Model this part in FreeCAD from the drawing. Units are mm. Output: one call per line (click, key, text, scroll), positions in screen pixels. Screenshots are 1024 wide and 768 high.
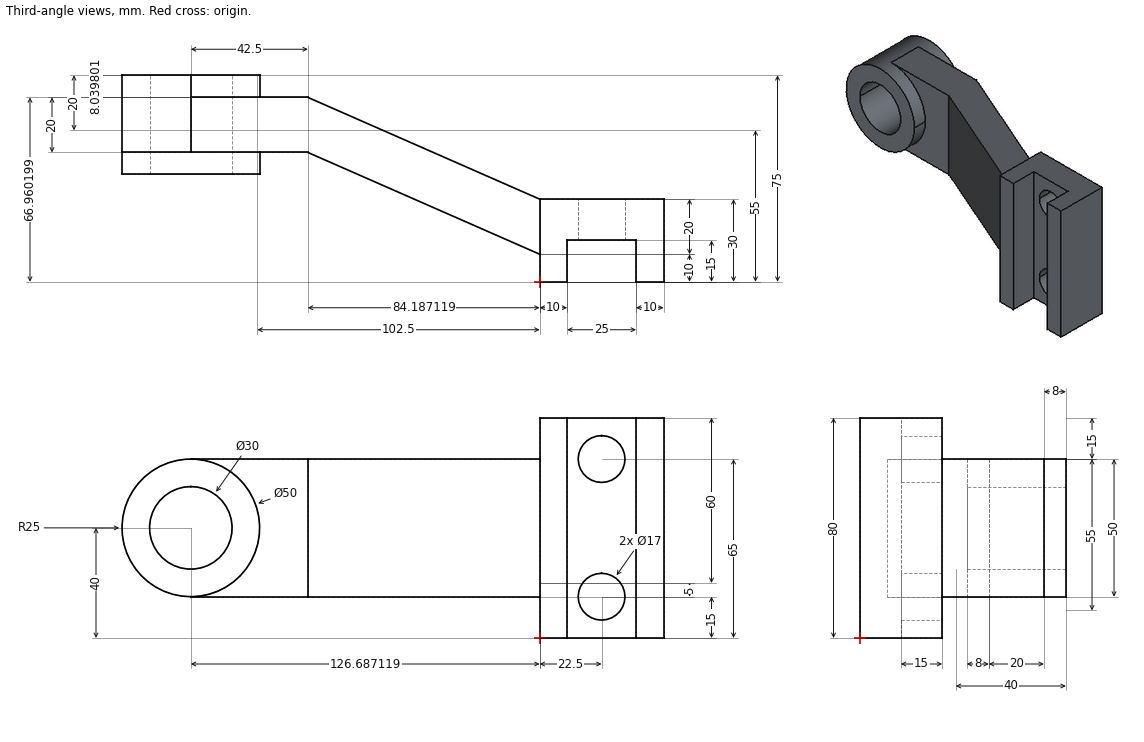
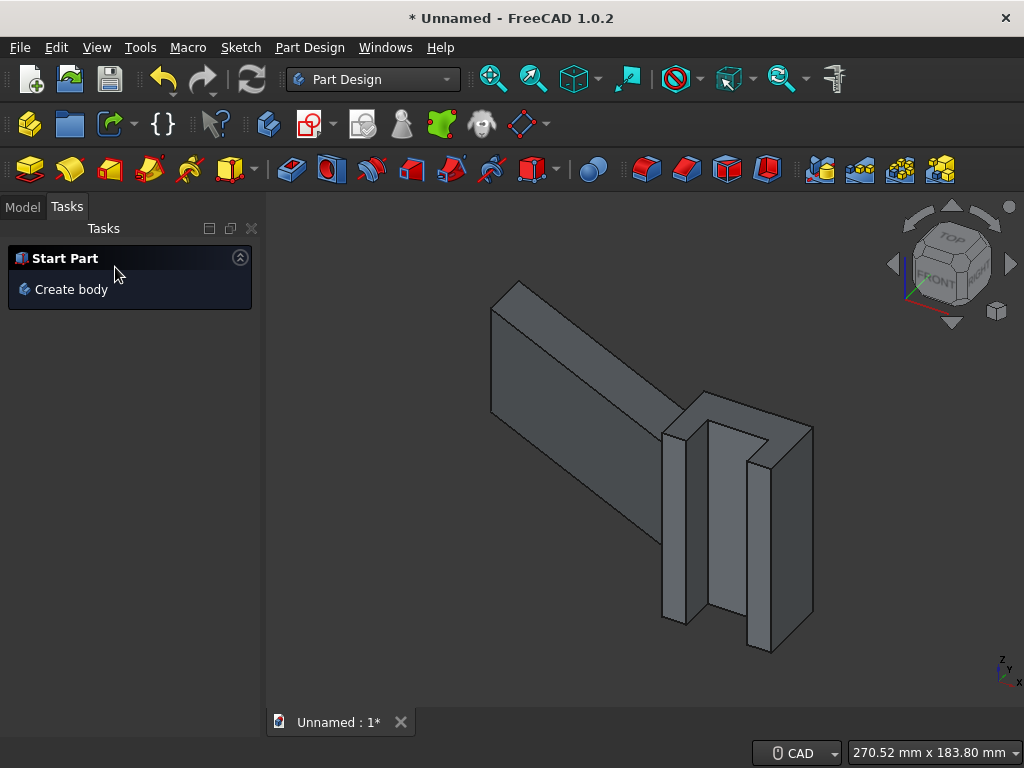
key(5)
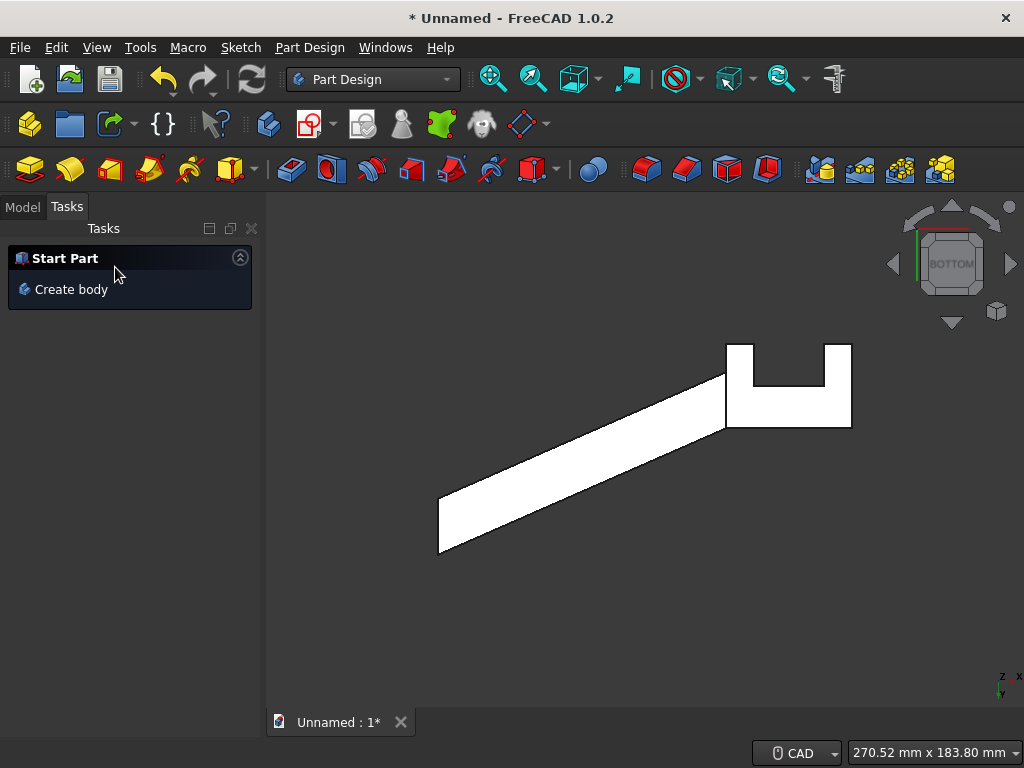
click(582, 463)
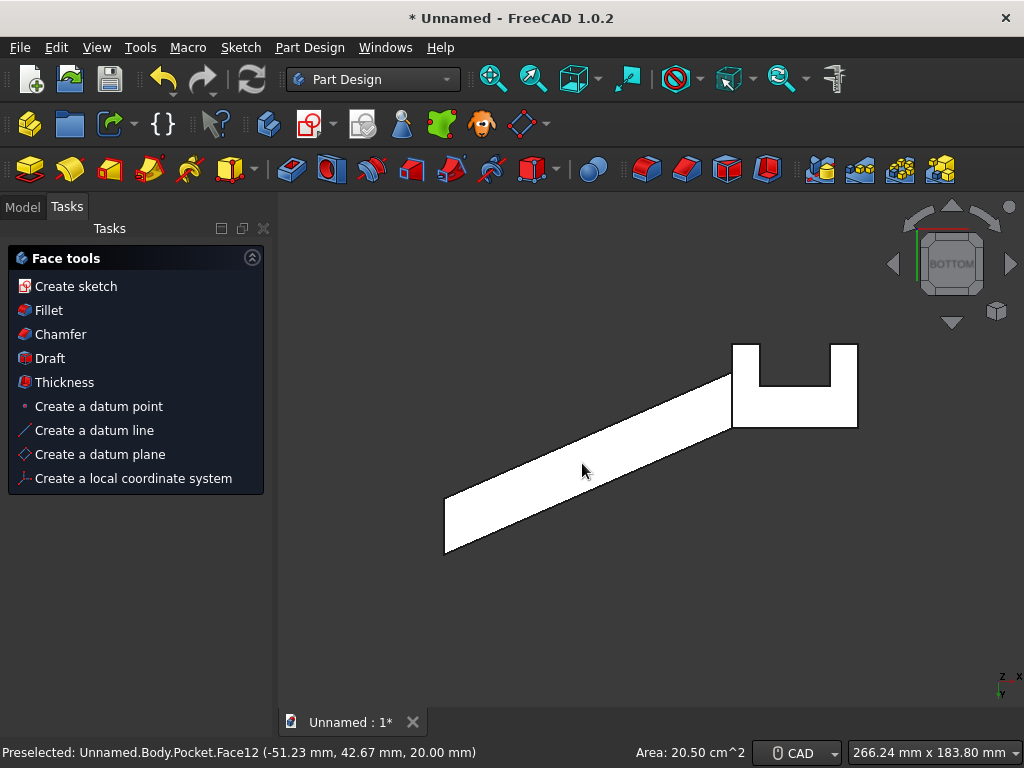
click(310, 124)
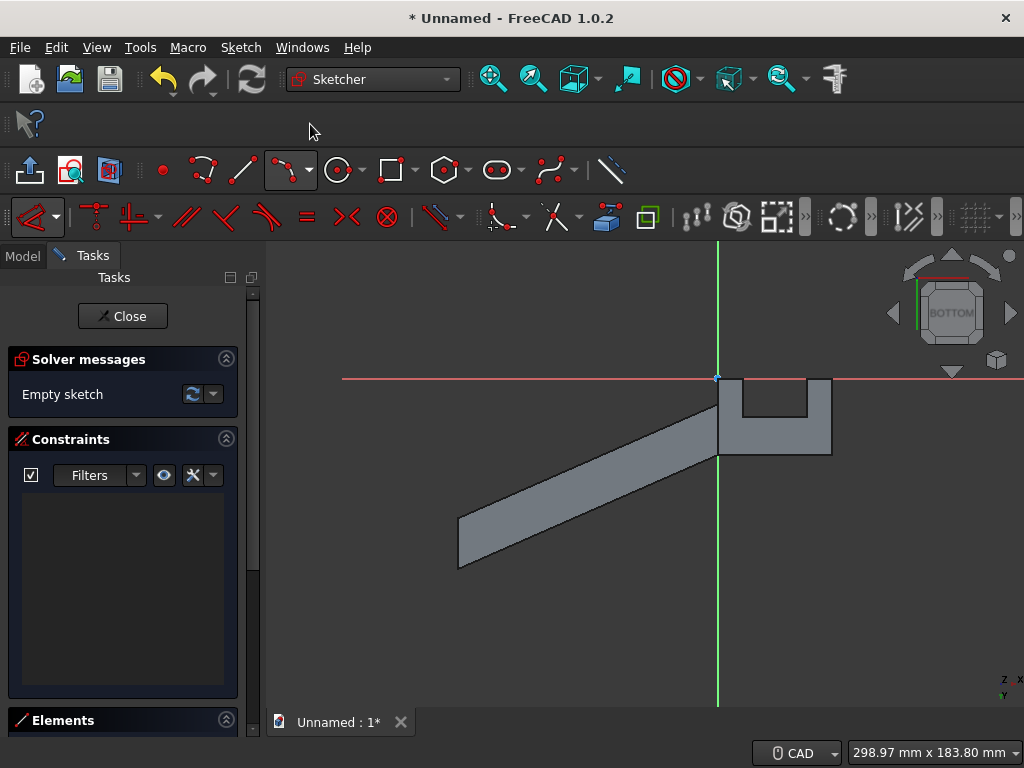
scroll(611, 474, up, 2)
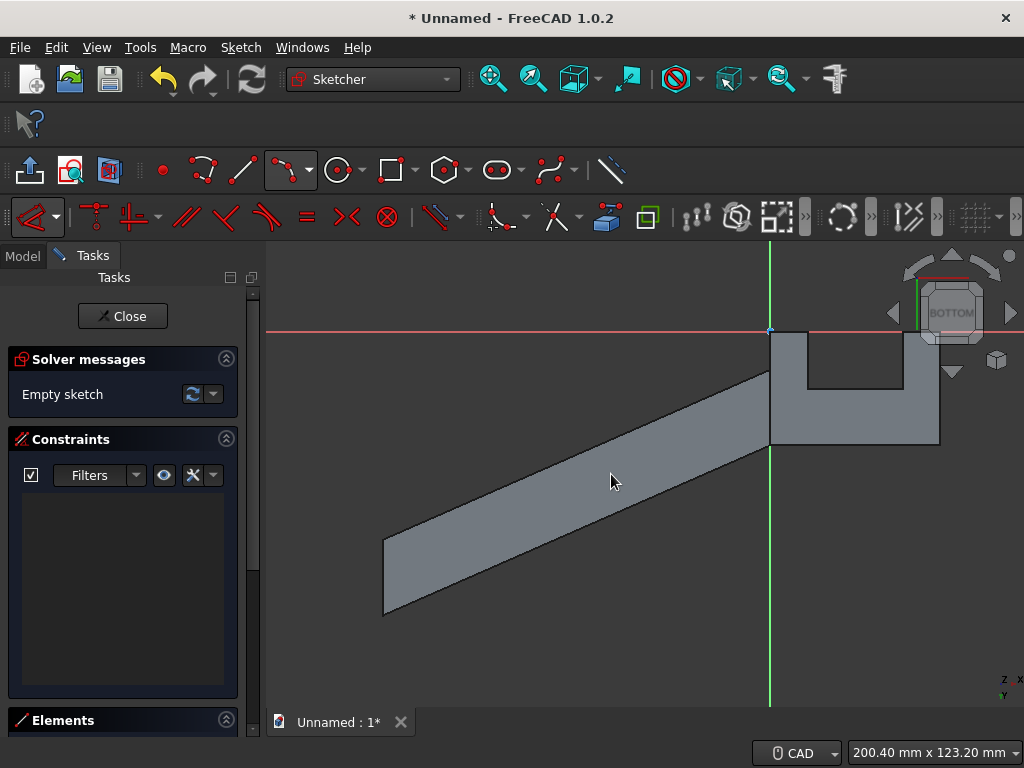
key(g)
key(m)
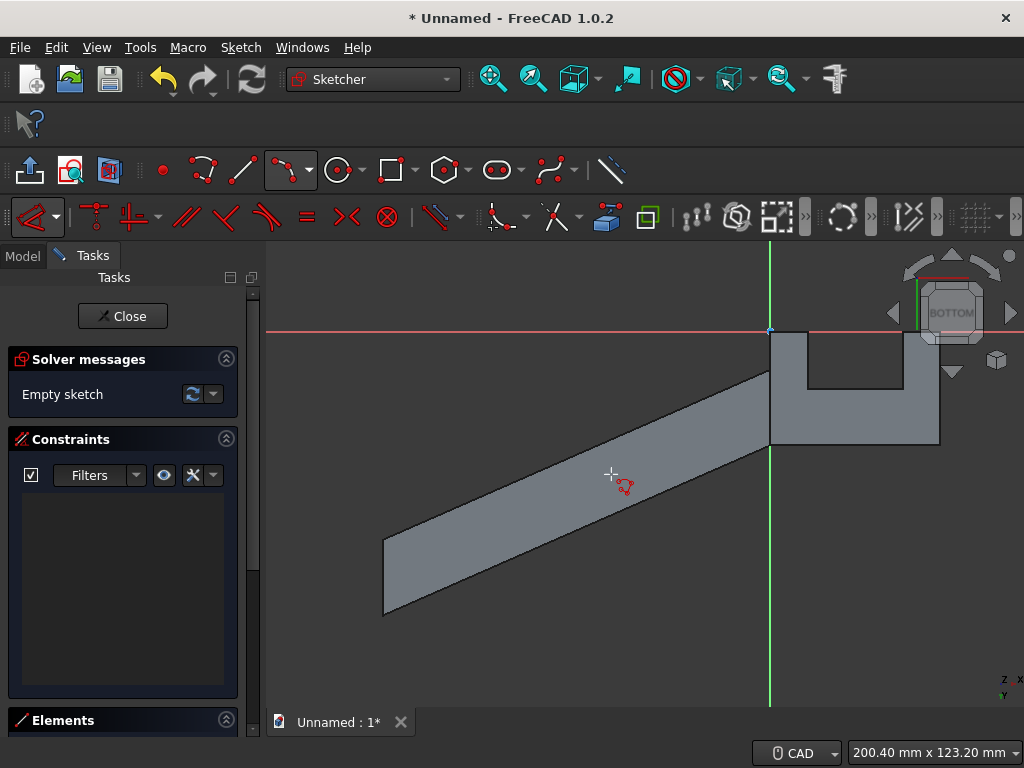
click(770, 370)
click(383, 540)
click(383, 616)
click(761, 445)
click(770, 371)
key(Escape)
key(Escape)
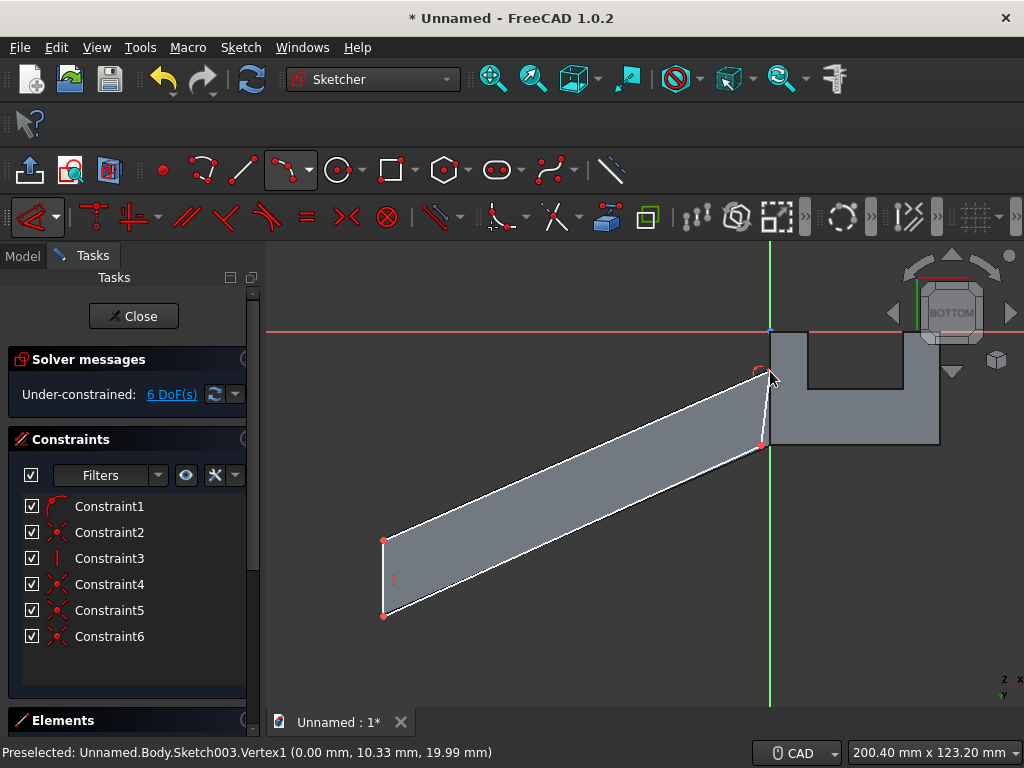
click(767, 393)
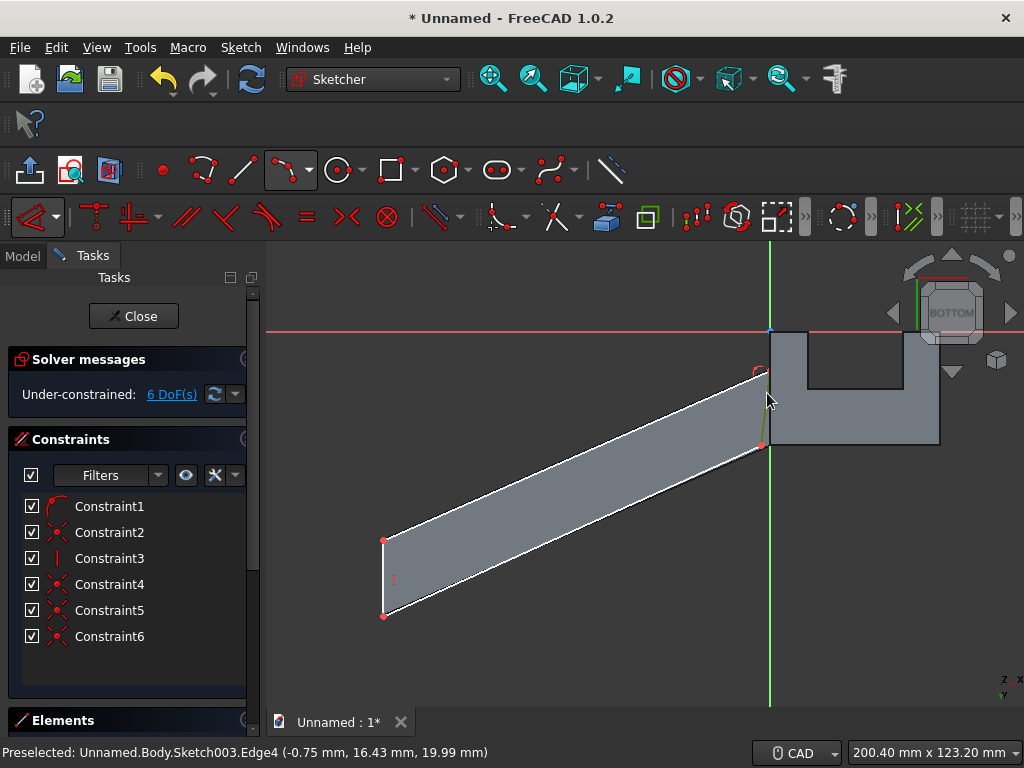
key(v)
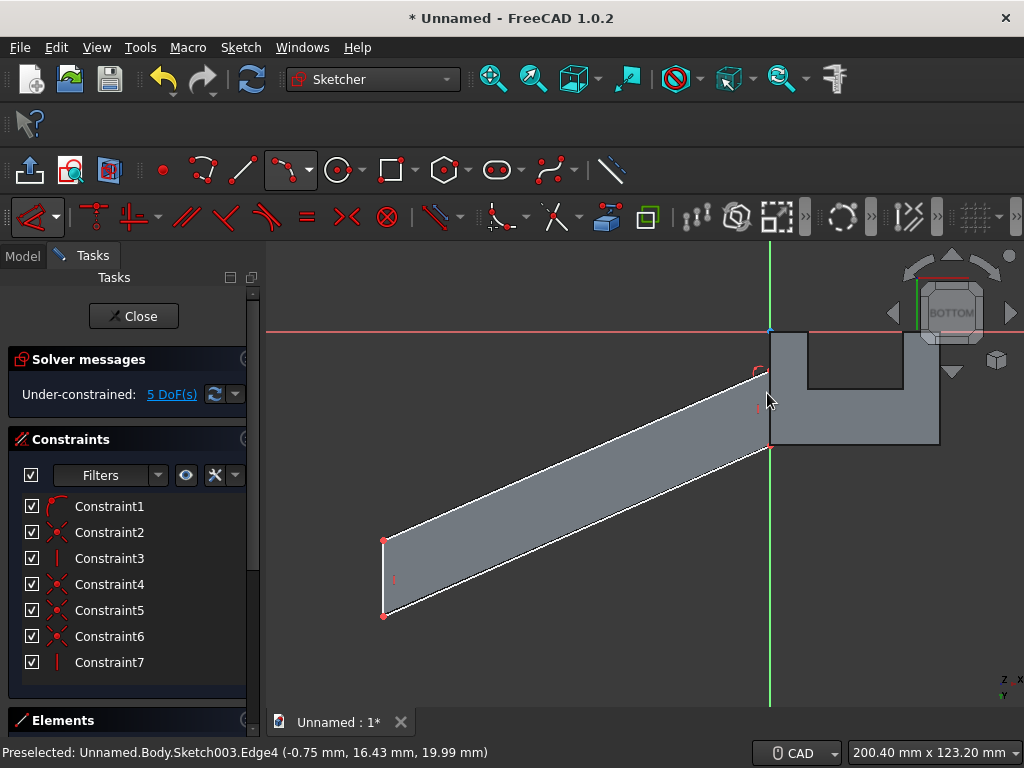
click(383, 564)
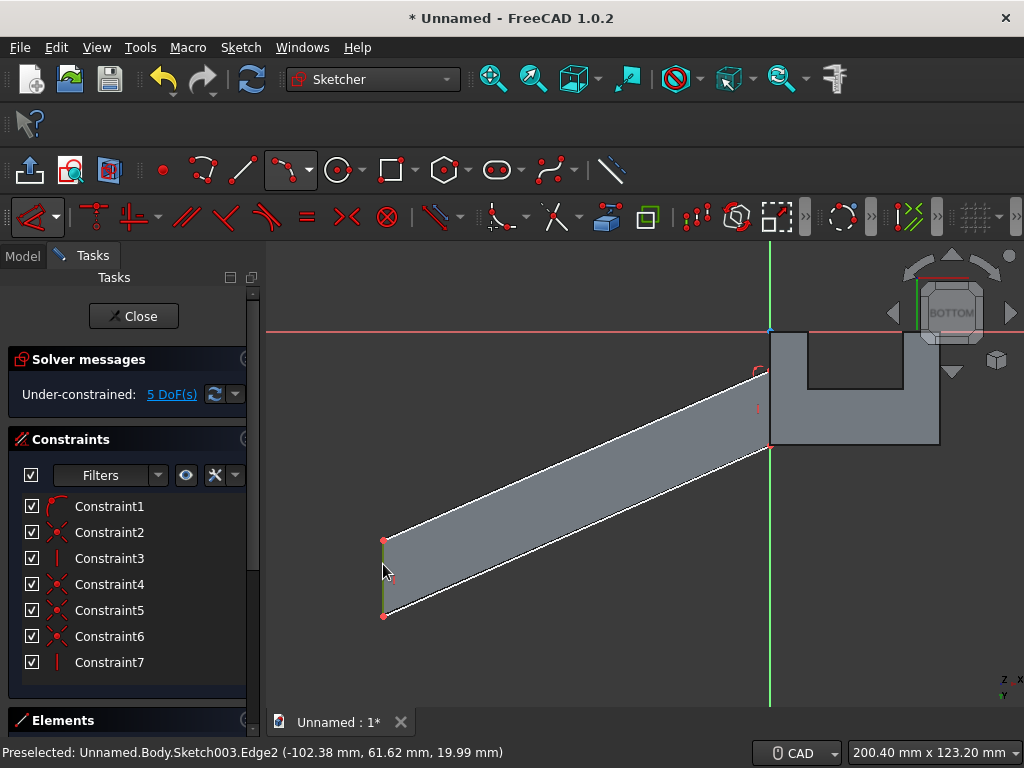
key(i)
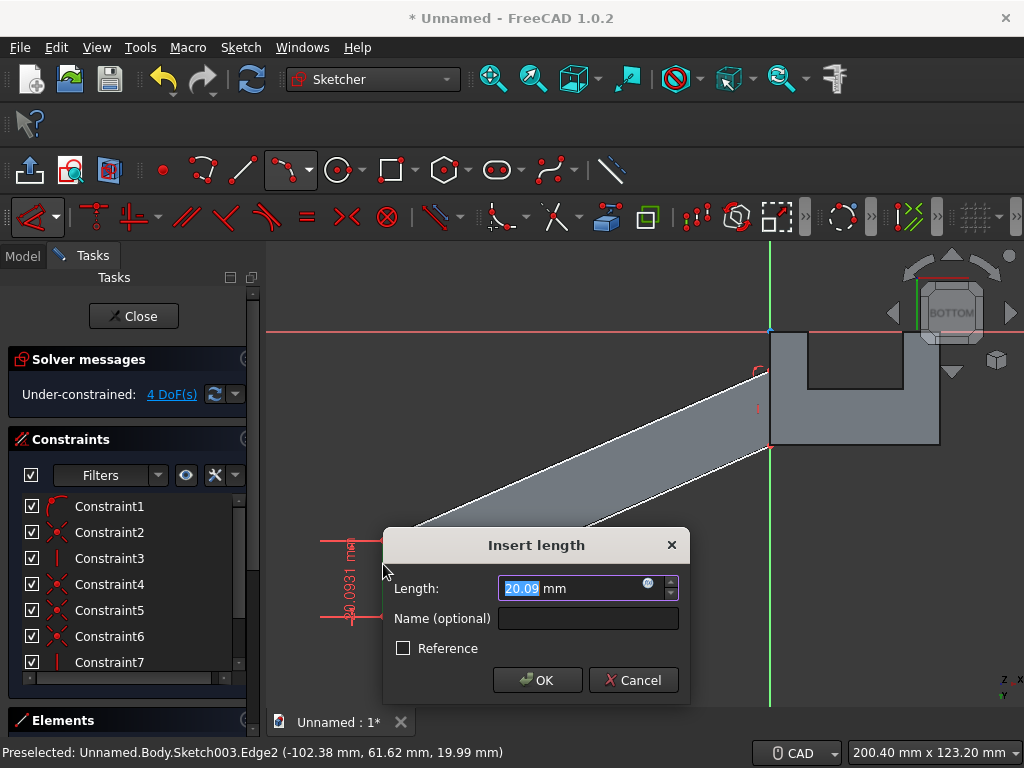
text(20)
key(Return)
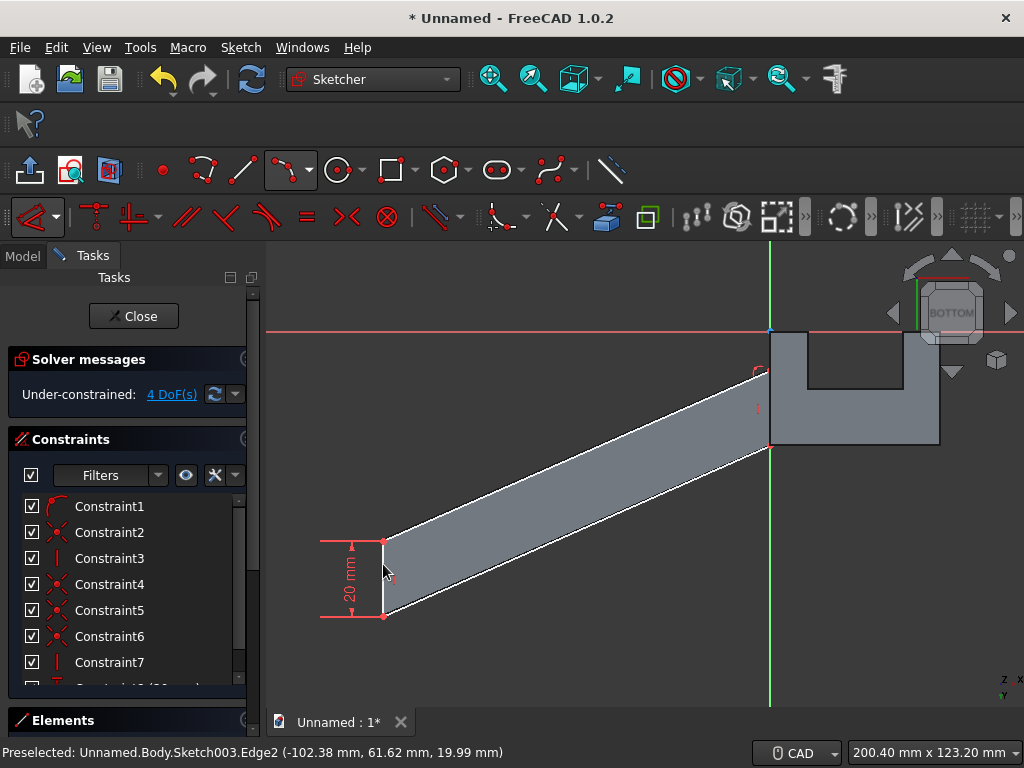
click(770, 423)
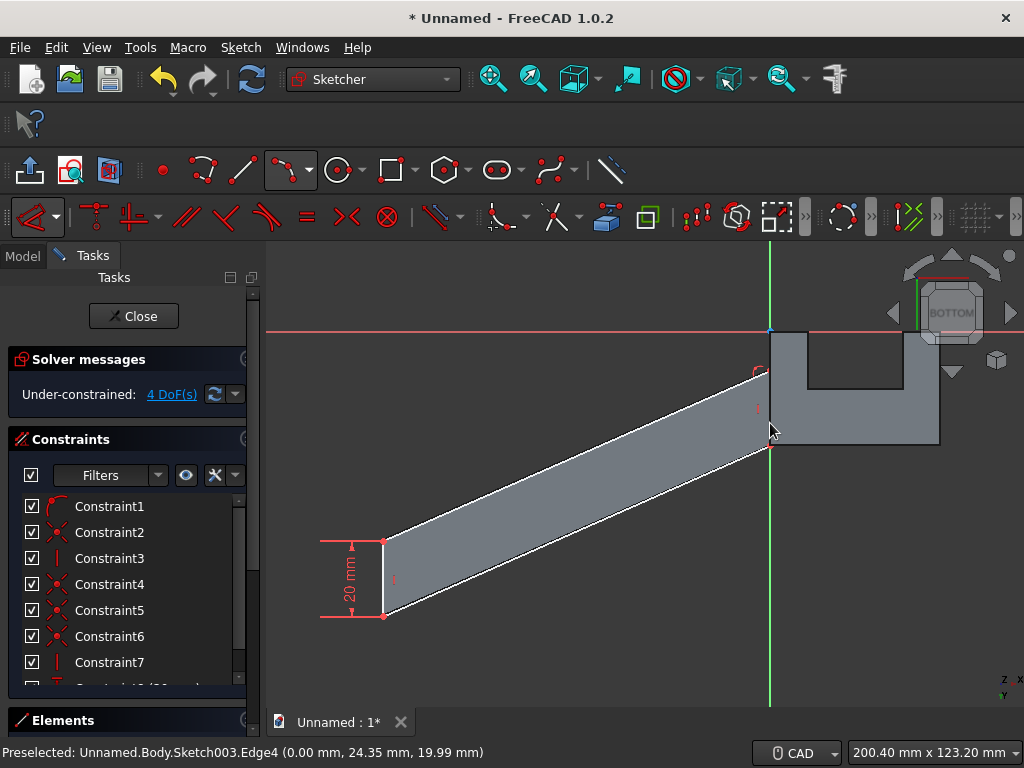
key(i)